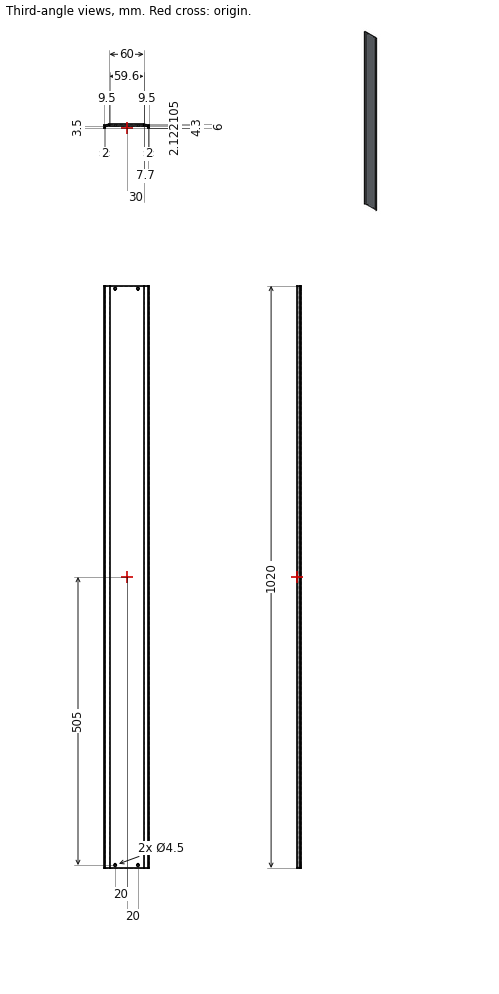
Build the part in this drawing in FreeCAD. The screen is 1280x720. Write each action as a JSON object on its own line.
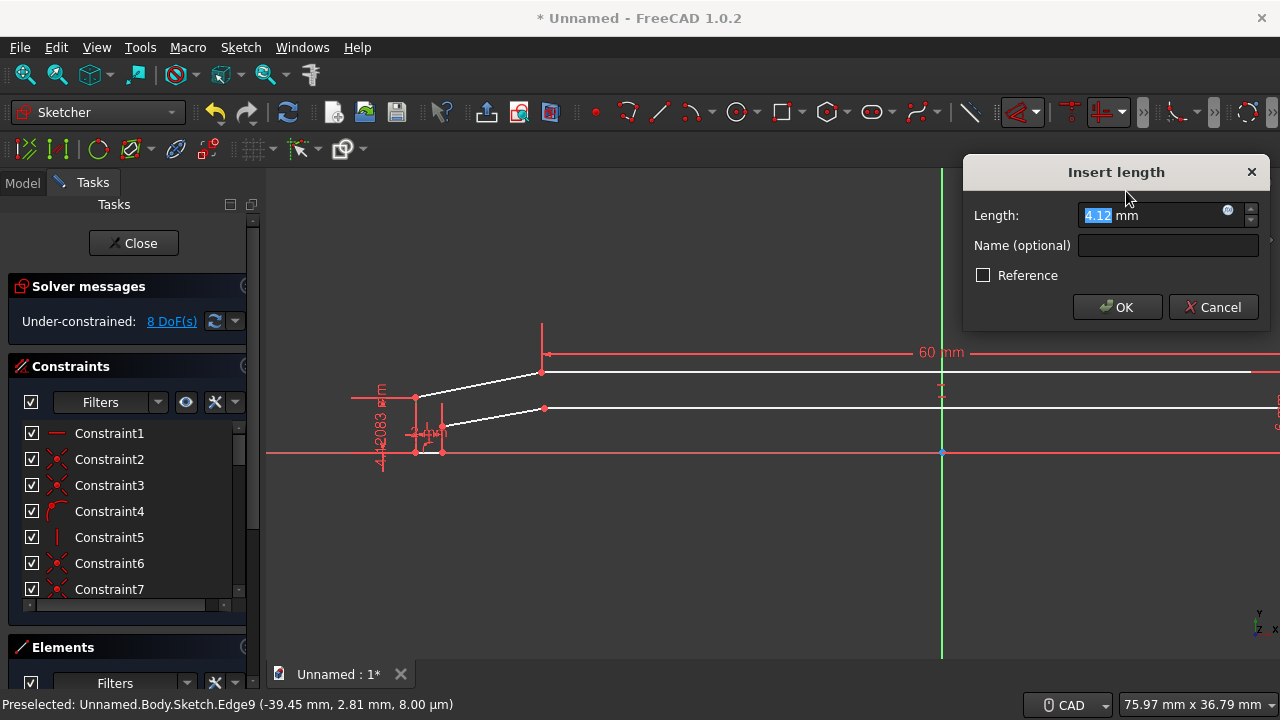
{"action": "type", "text": "4.3"}
{"action": "key", "text": "Return"}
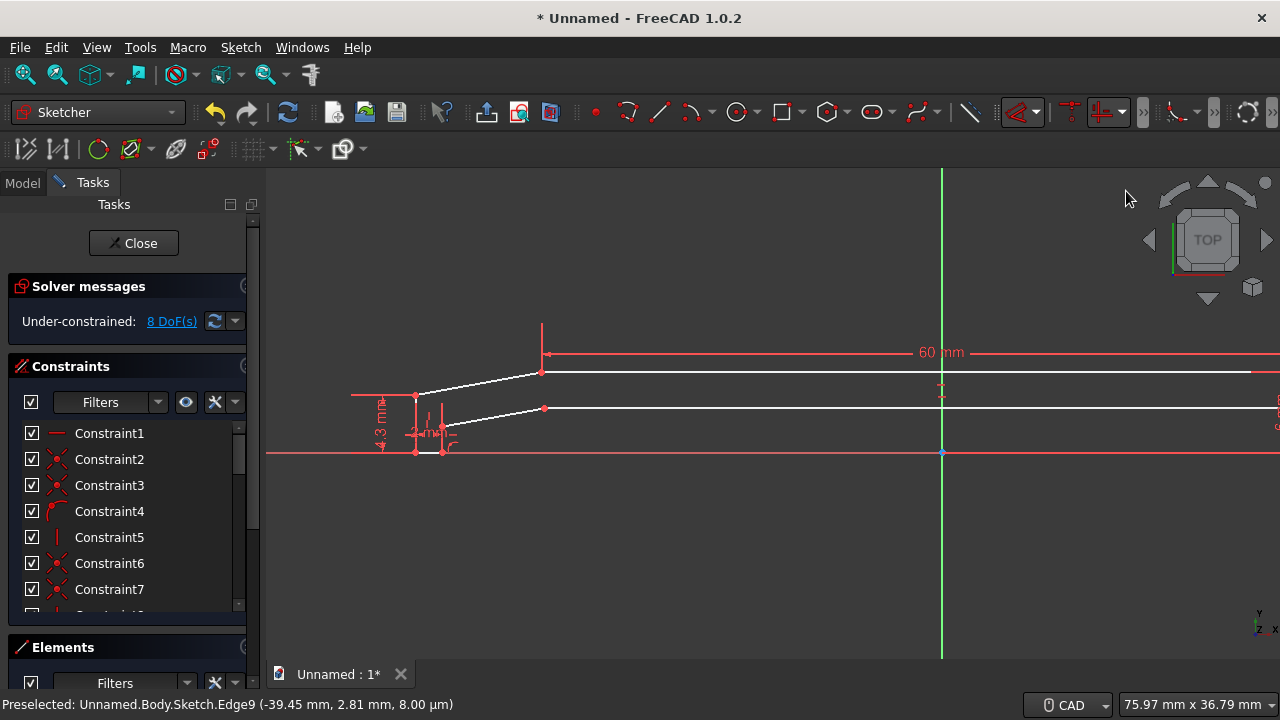
{"action": "scroll", "coordinate": [416, 415], "scroll_direction": "down", "scroll_amount": 3}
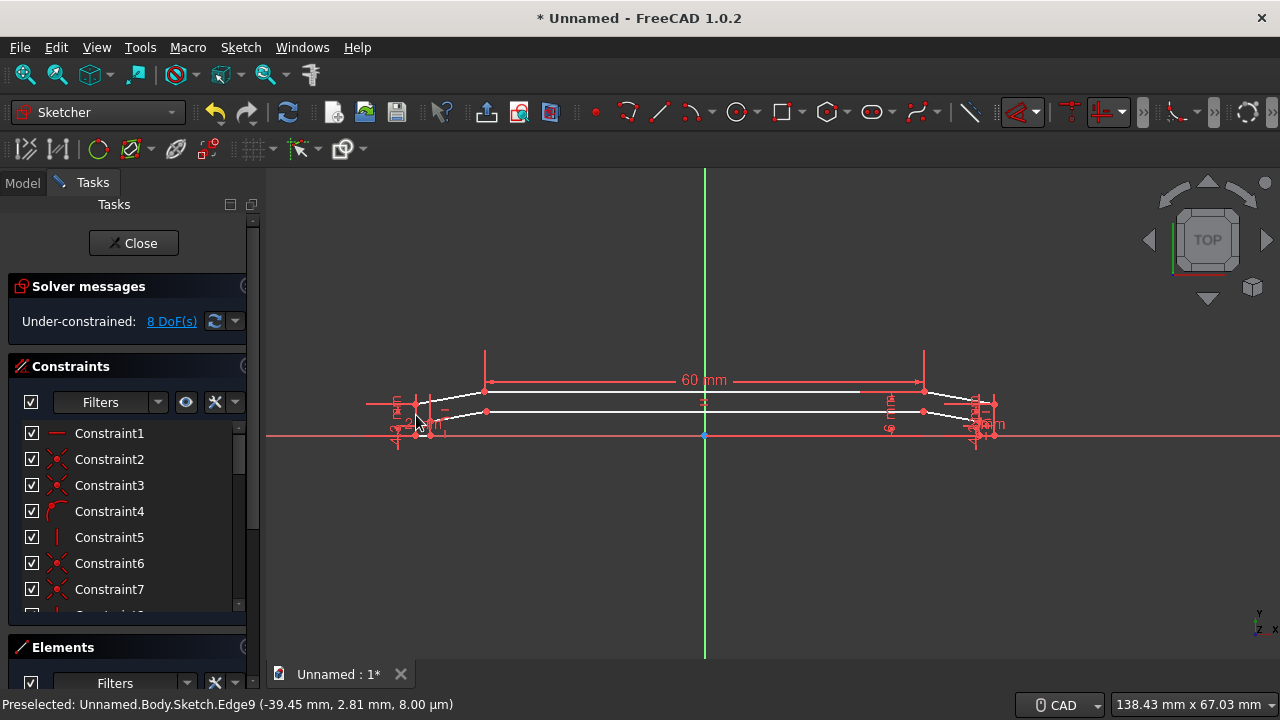
{"action": "left_click", "coordinate": [924, 392]}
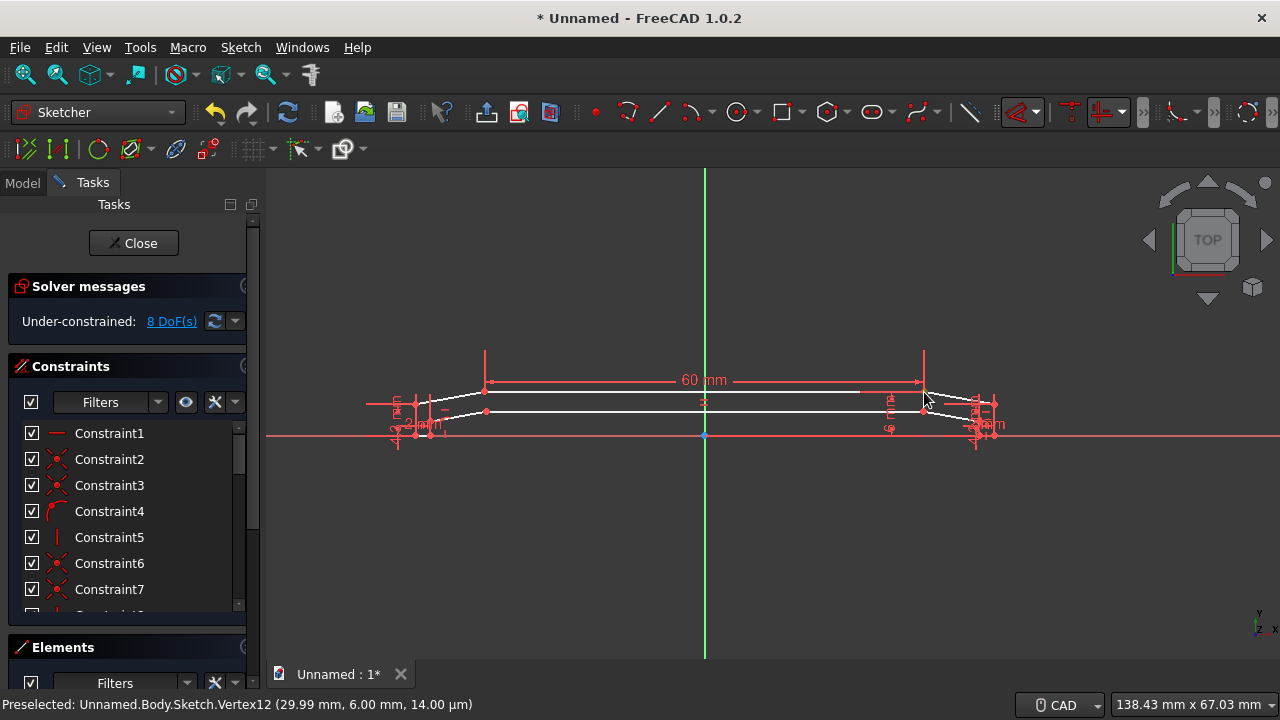
{"action": "key", "text": "l"}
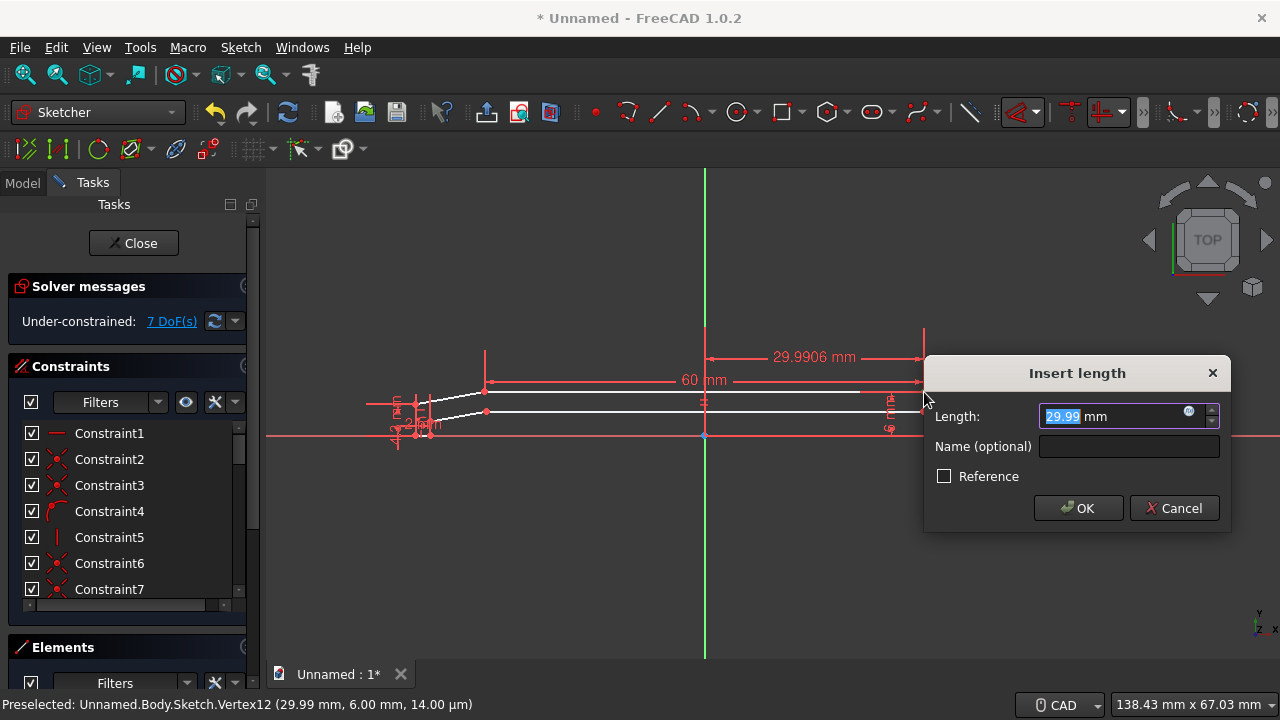
{"action": "type", "text": "30"}
{"action": "key", "text": "Return"}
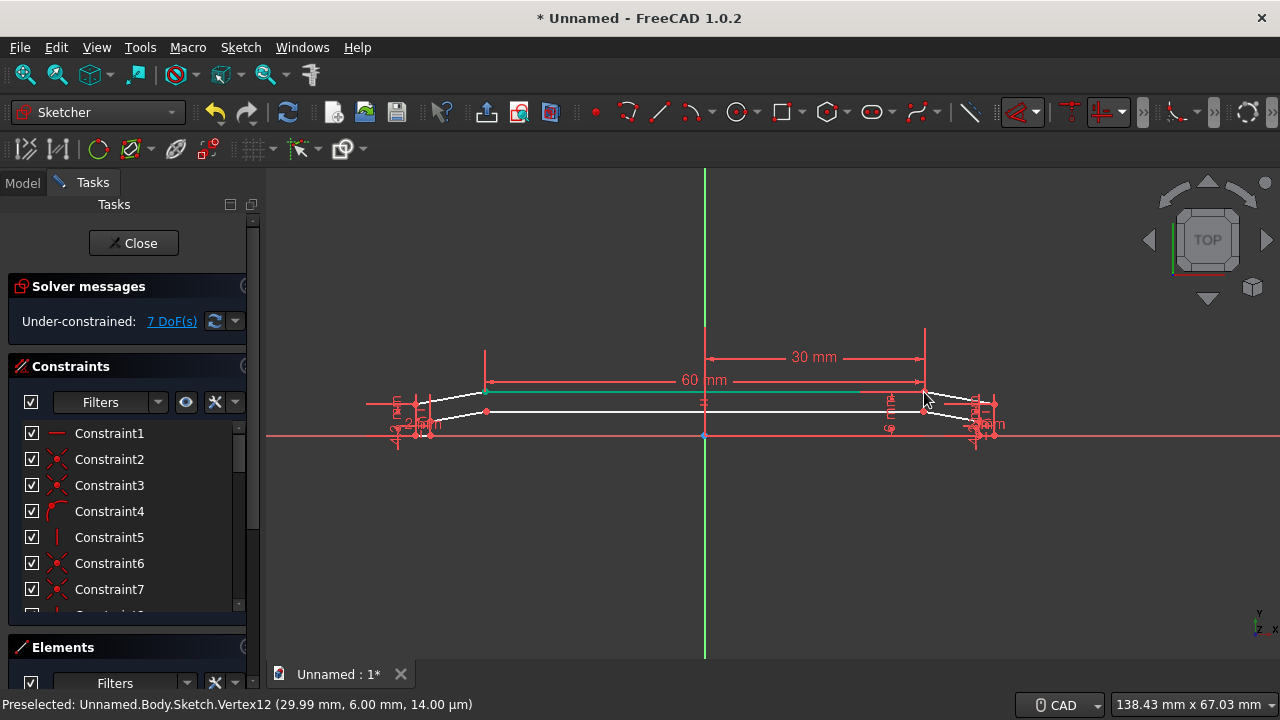
{"action": "left_click", "coordinate": [618, 412]}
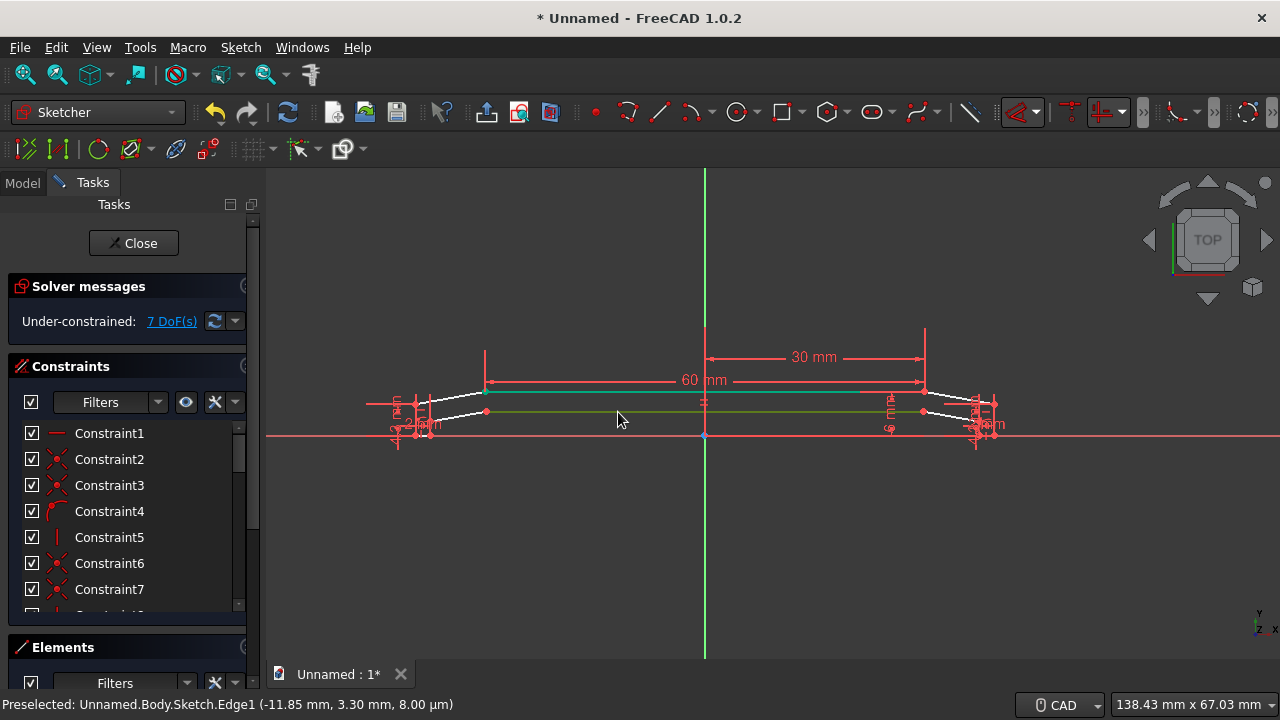
{"action": "left_click", "coordinate": [1038, 112]}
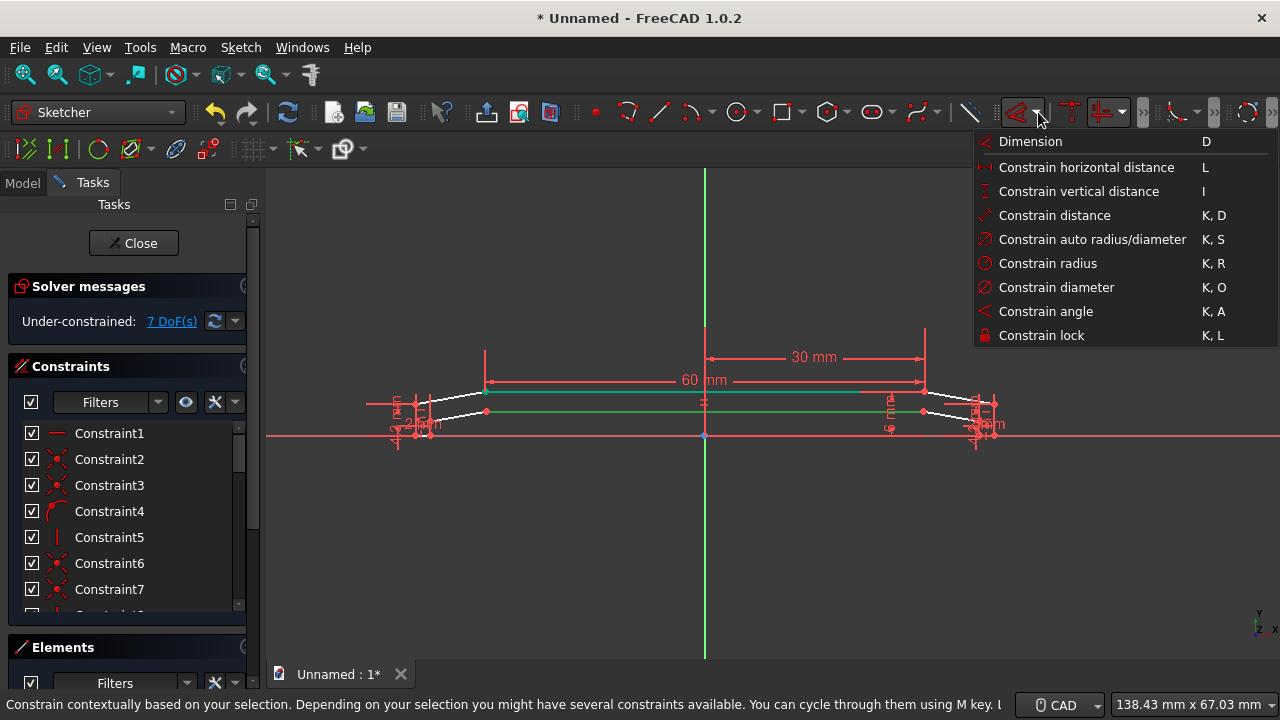
{"action": "left_click", "coordinate": [1126, 167]}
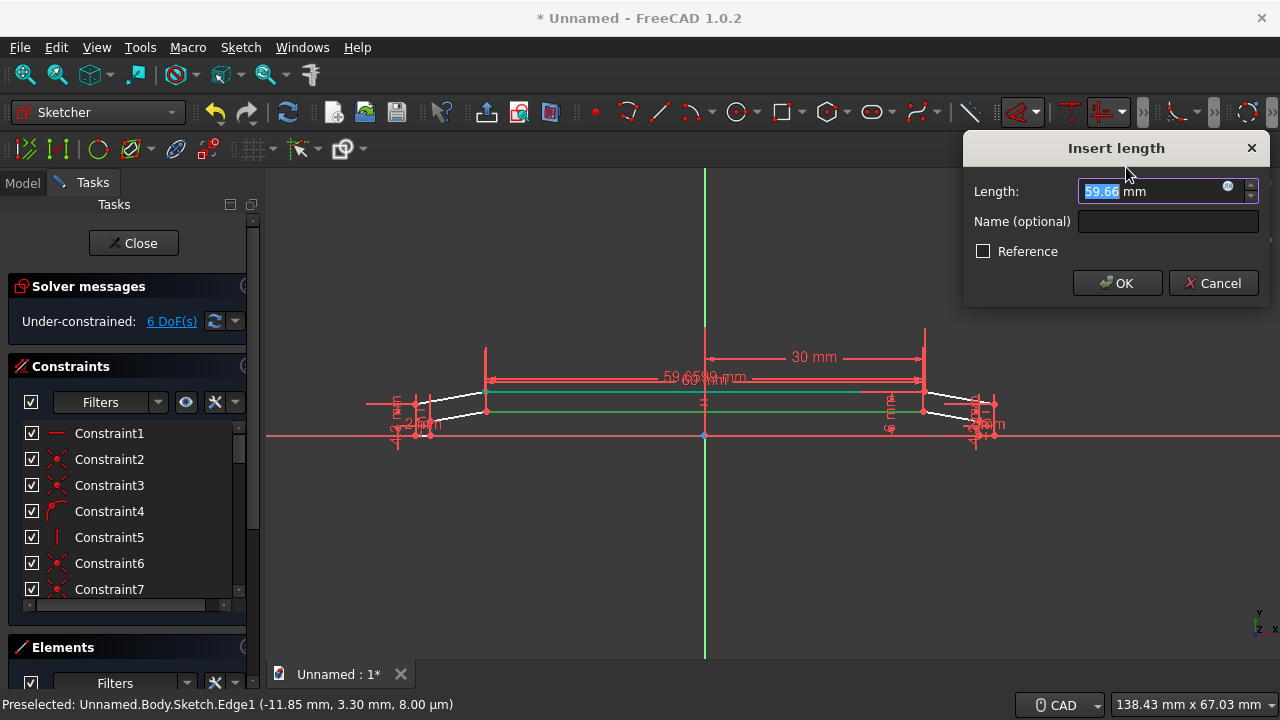
{"action": "type", "text": "59.6"}
{"action": "key", "text": "Return"}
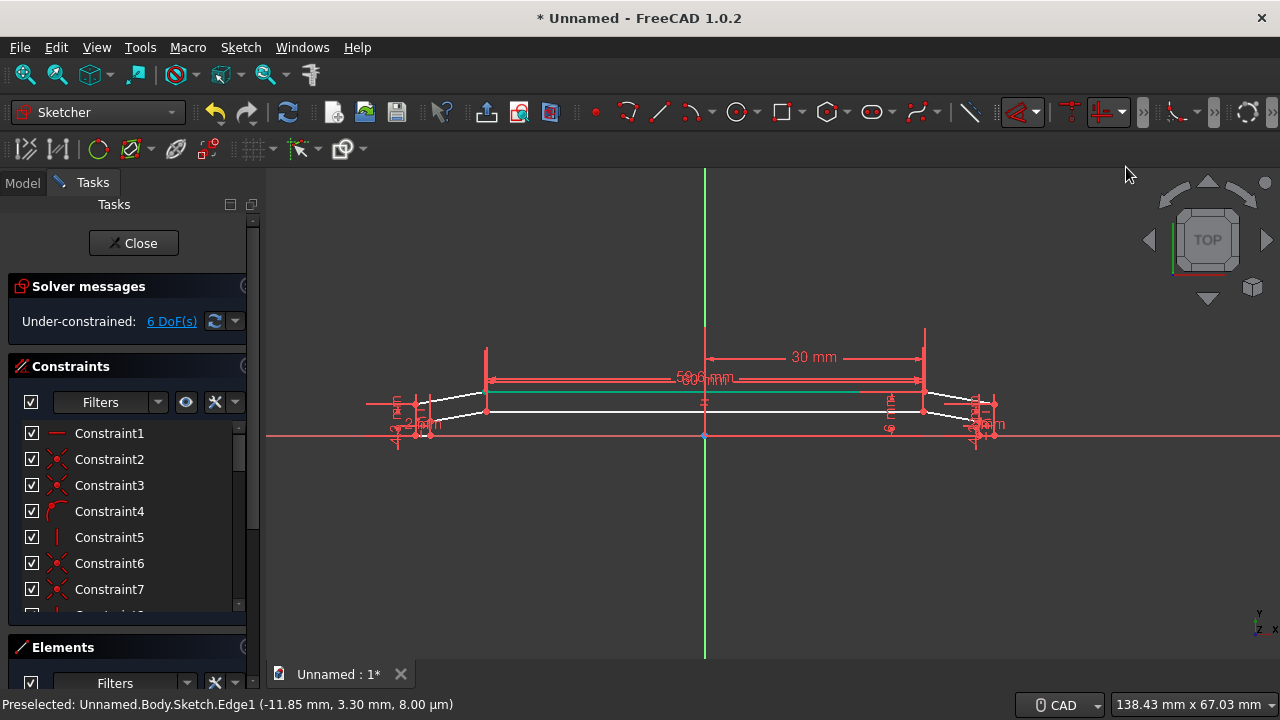
{"action": "scroll", "coordinate": [487, 412], "scroll_direction": "up", "scroll_amount": 3}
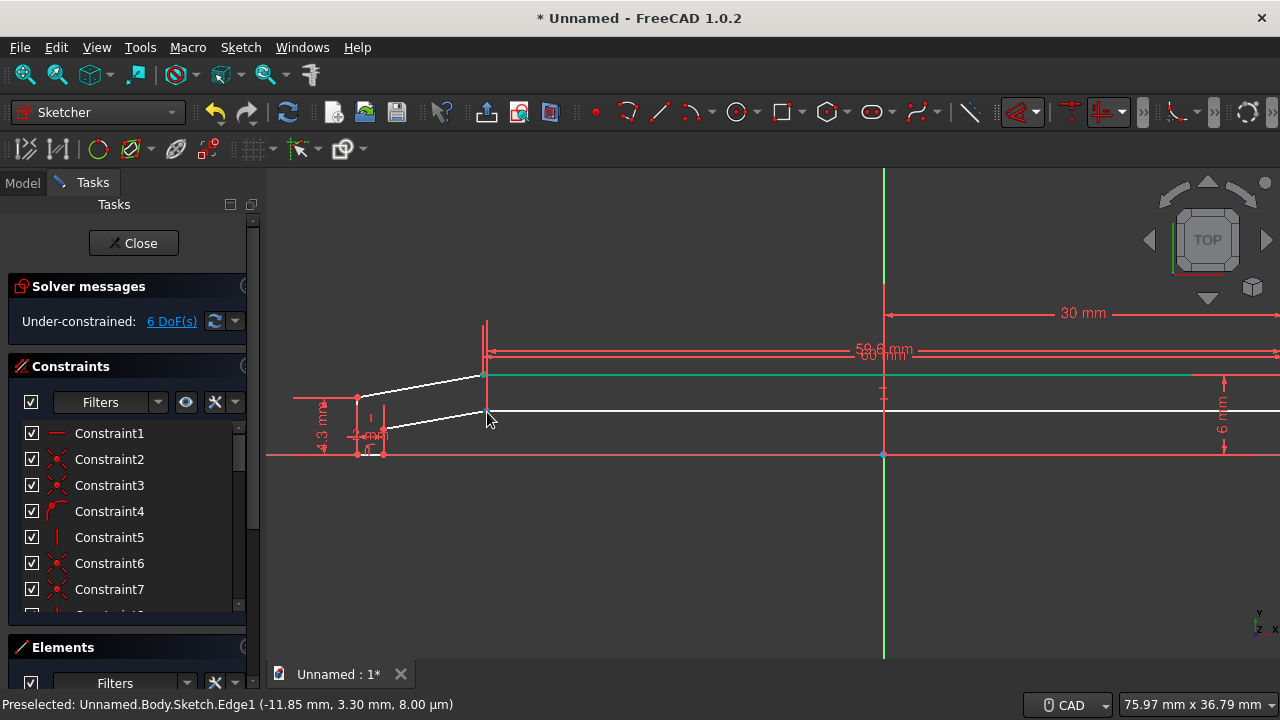
{"action": "left_click", "coordinate": [487, 411]}